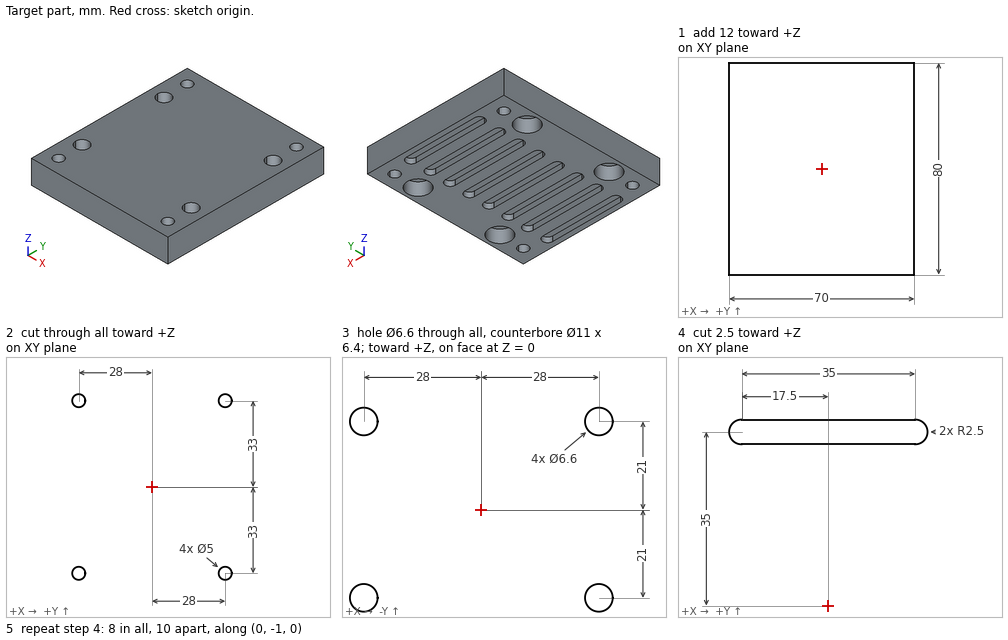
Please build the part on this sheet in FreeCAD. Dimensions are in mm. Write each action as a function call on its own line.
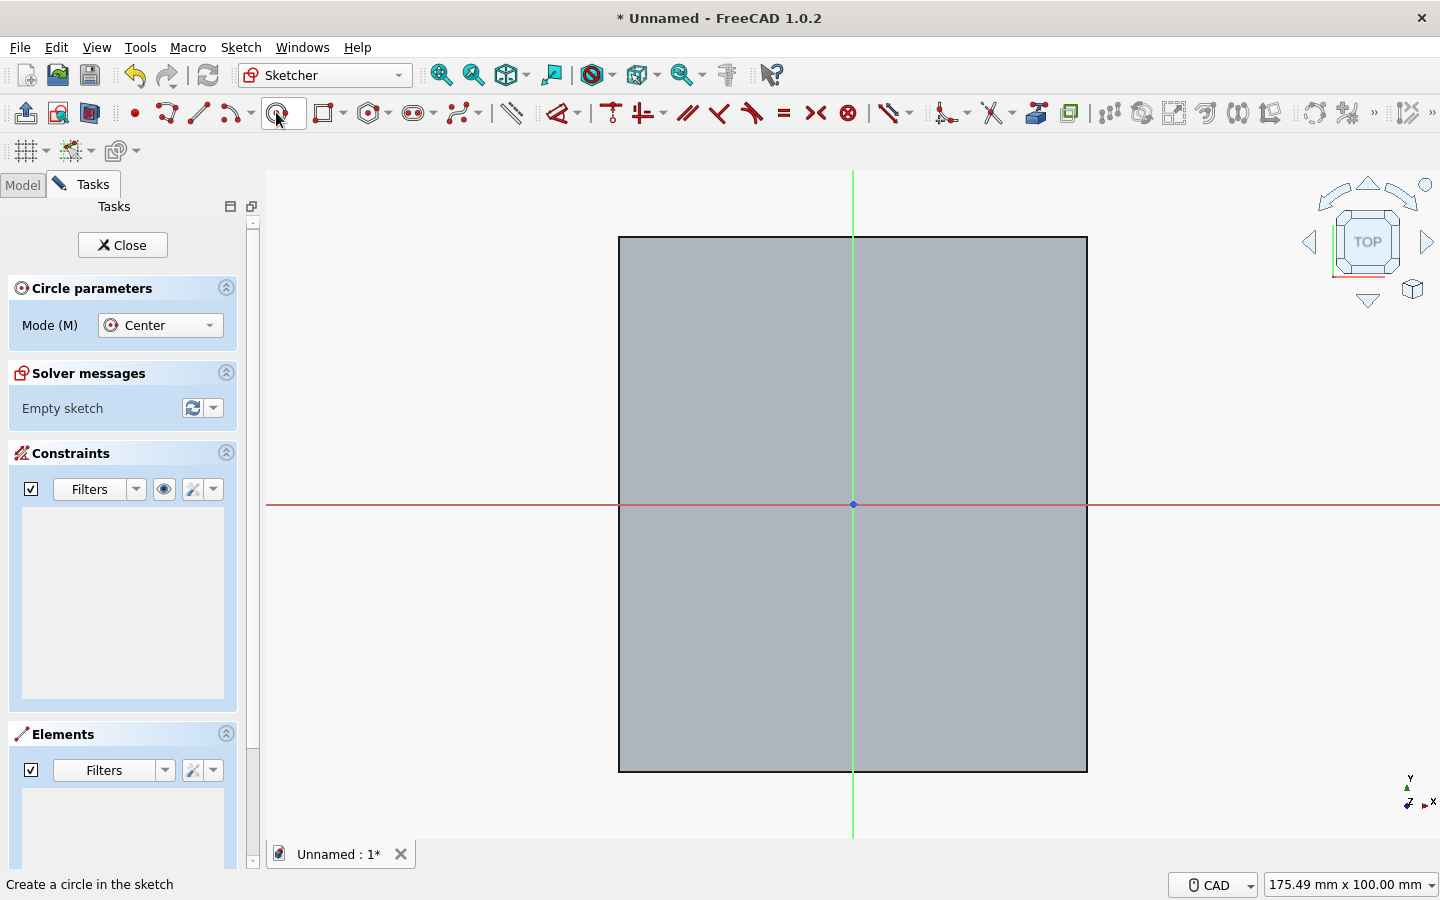
scroll(1040, 725, up, 2)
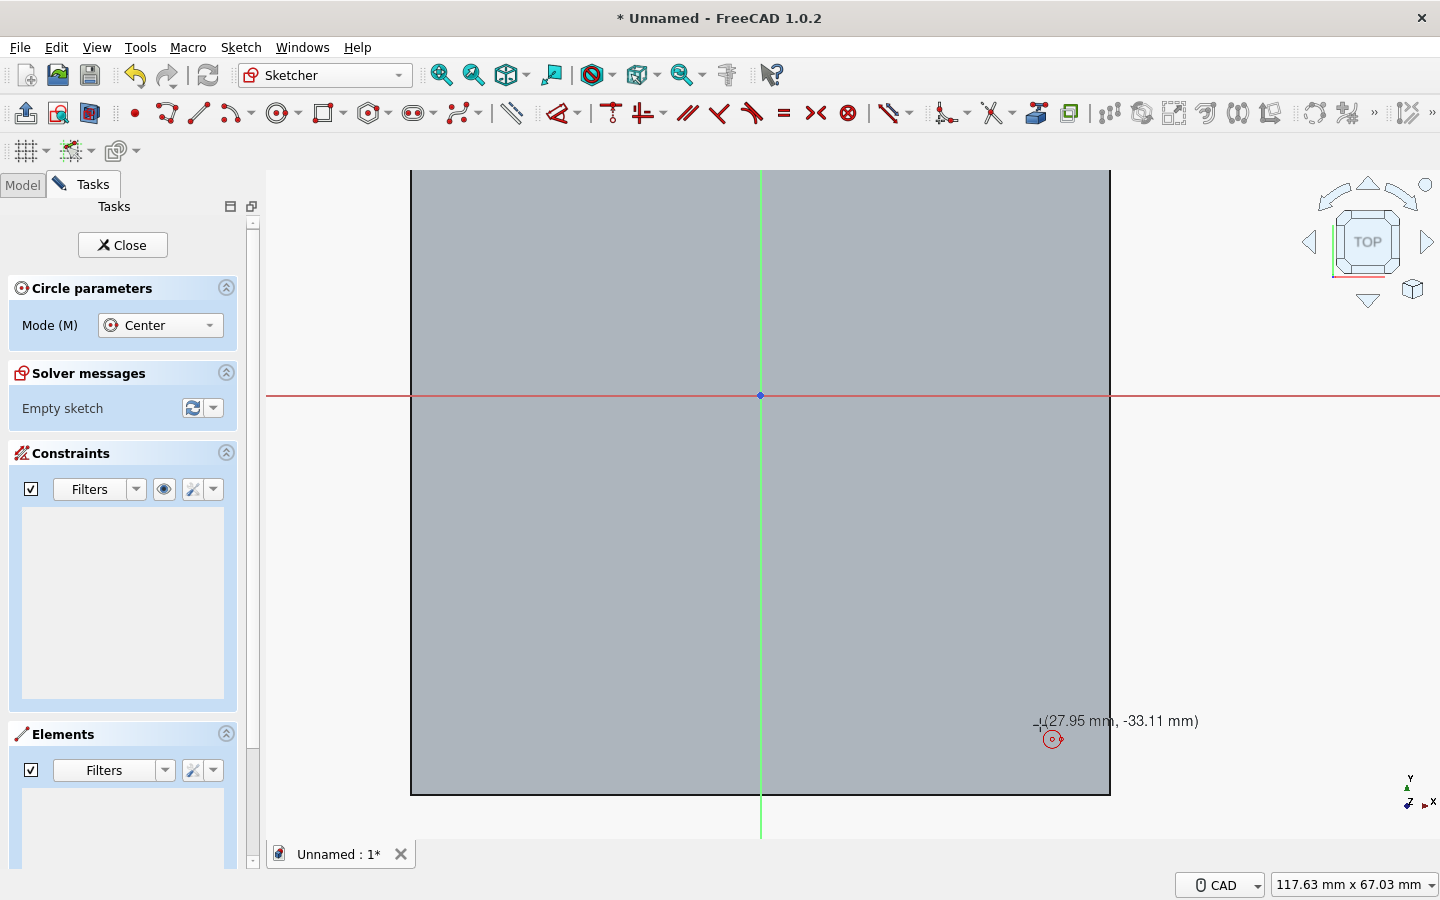
click(1040, 725)
move(1058, 707)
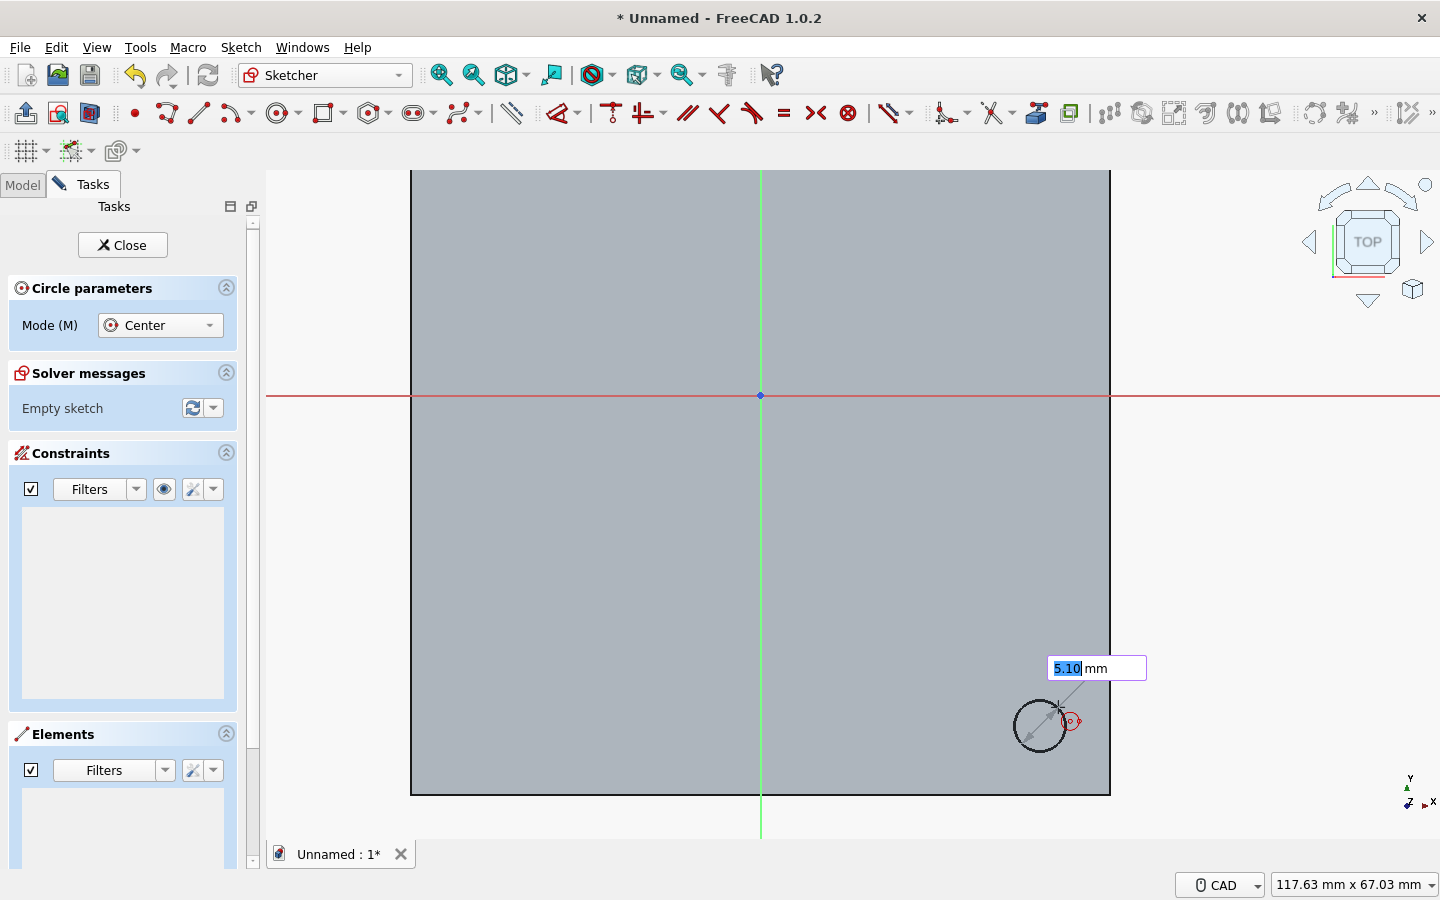
text(5)
key(Return)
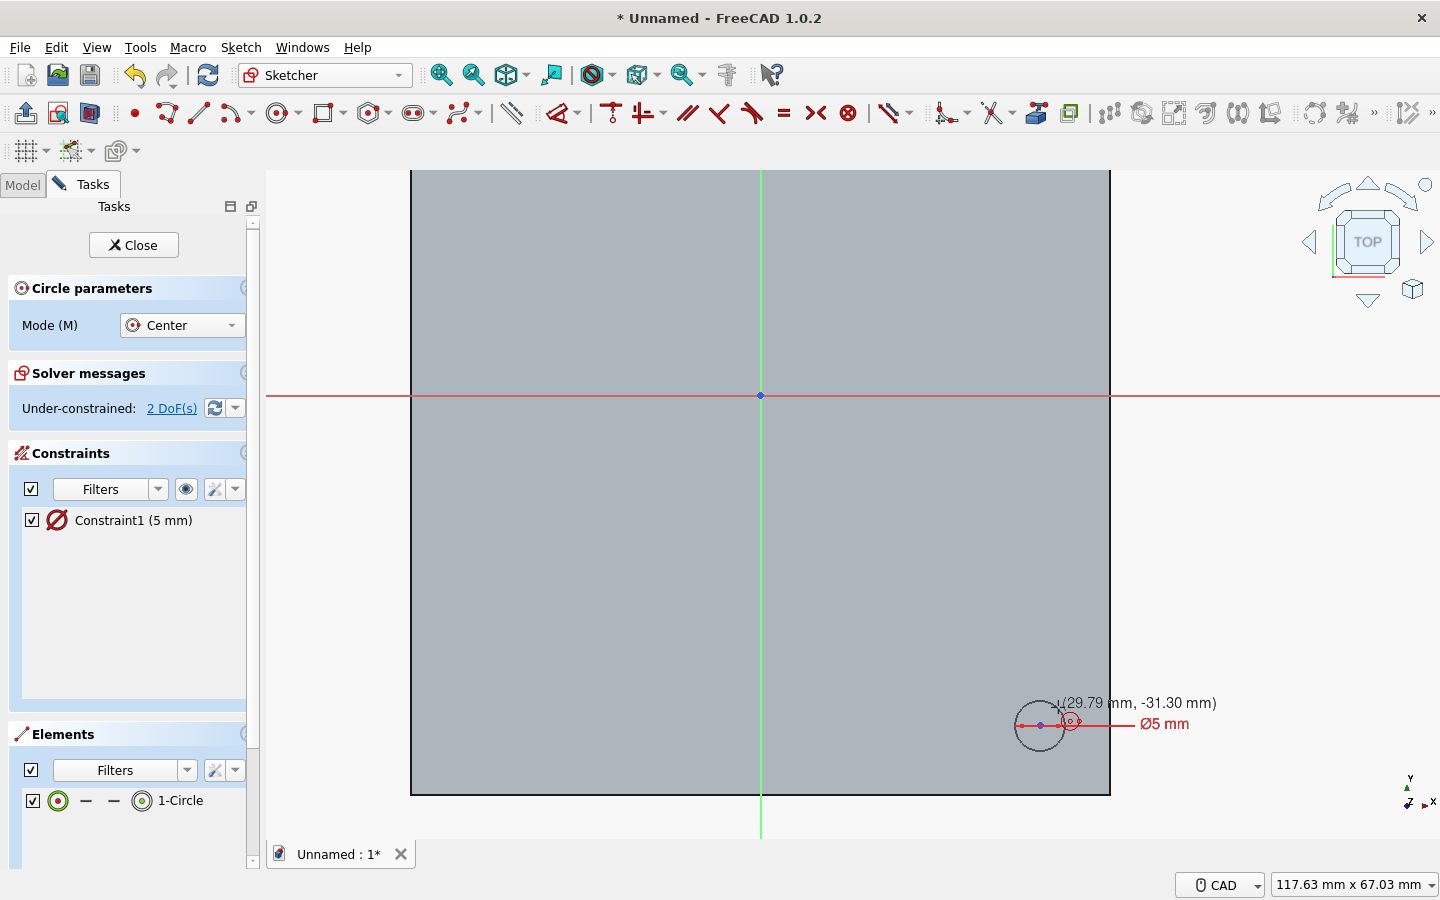
scroll(833, 726, down, 2)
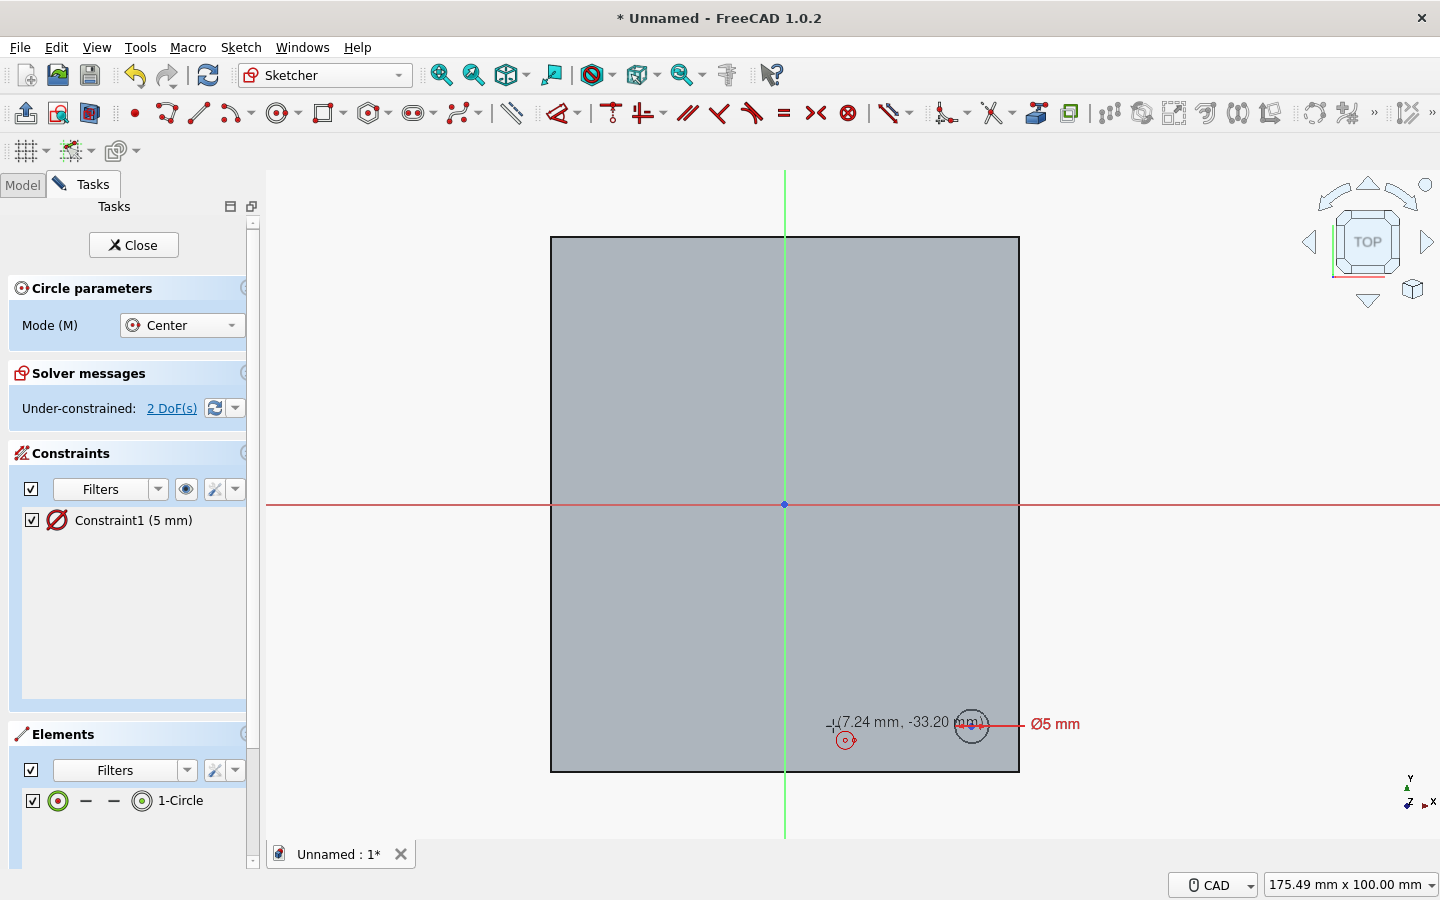
scroll(972, 284, up, 2)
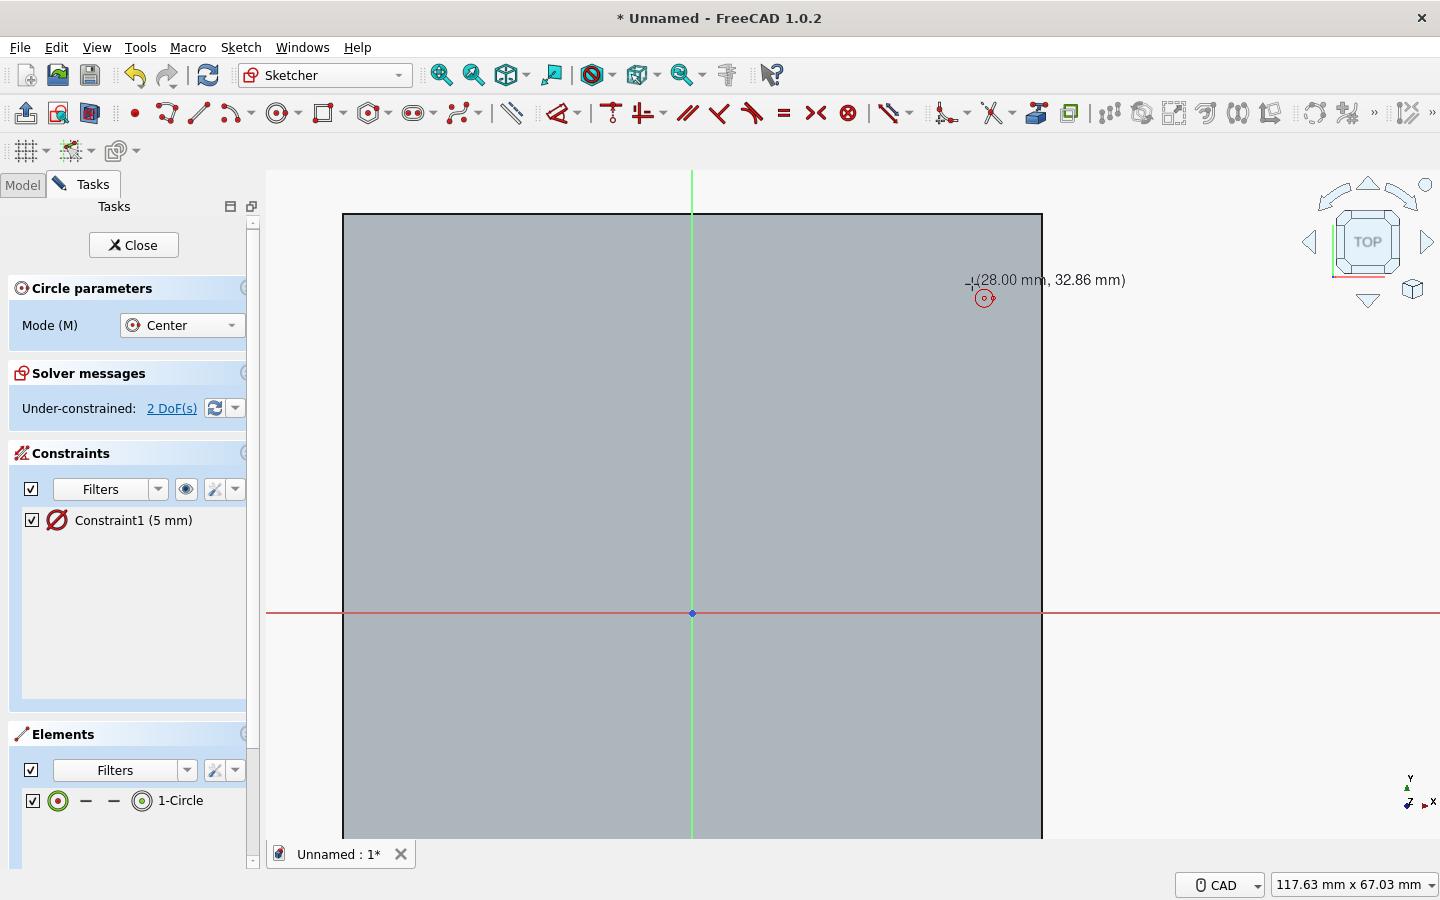
click(972, 284)
move(989, 266)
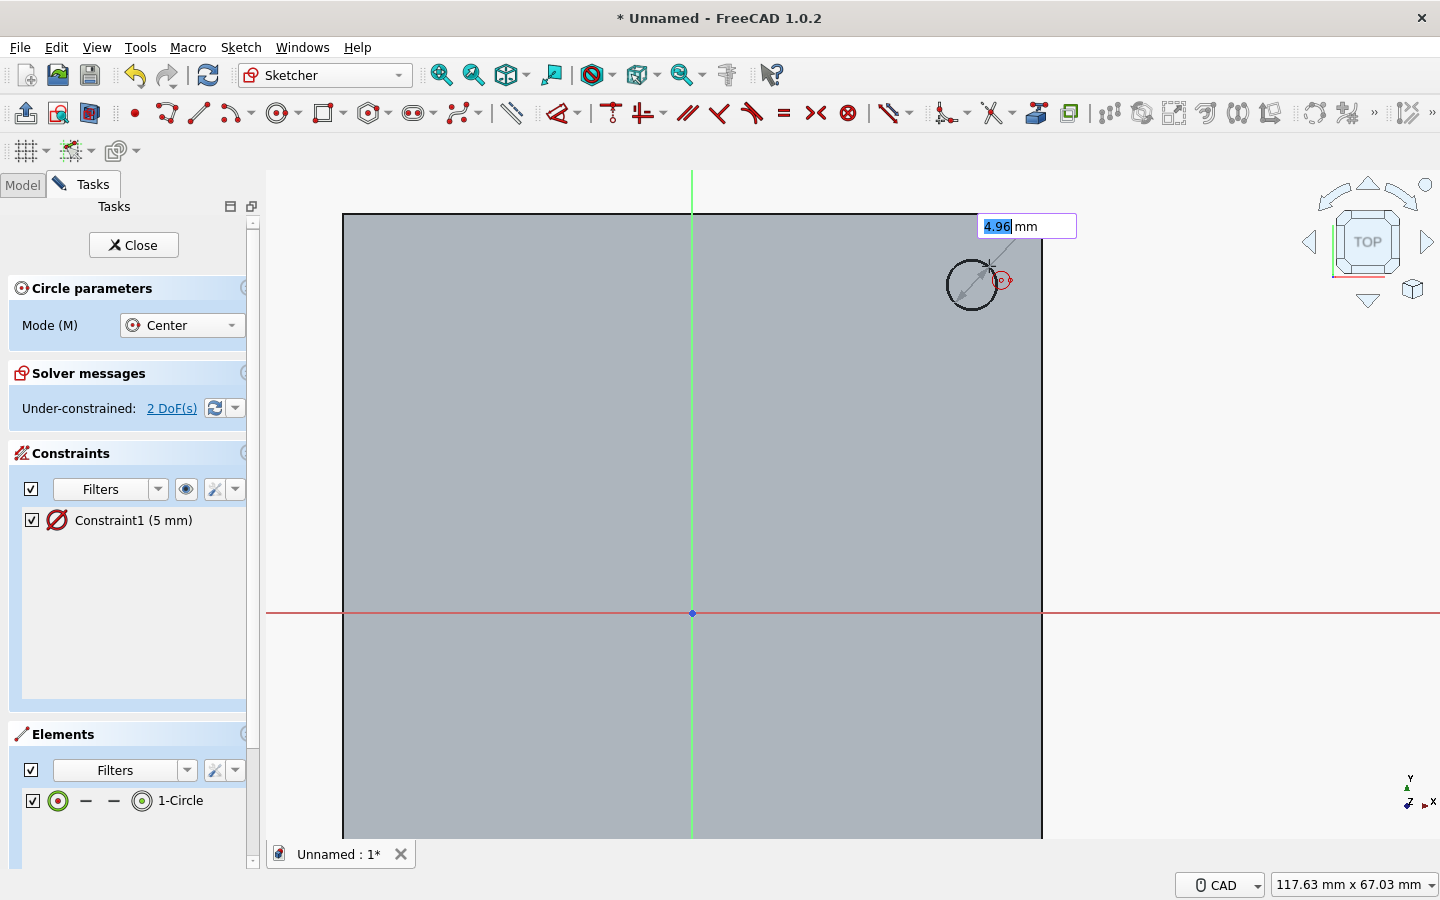
text(5)
key(Return)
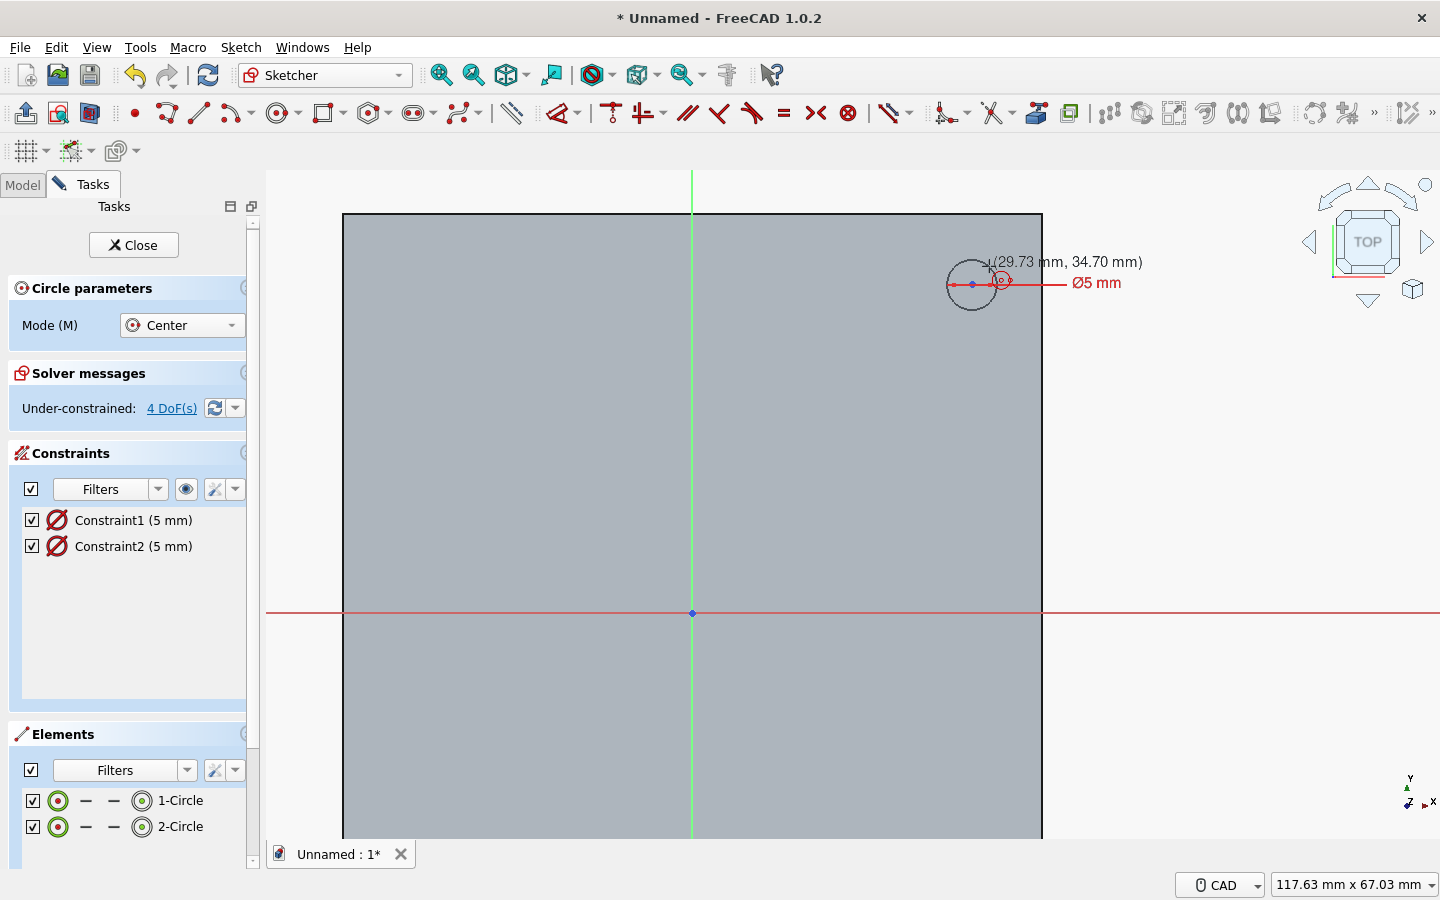
click(413, 284)
move(430, 266)